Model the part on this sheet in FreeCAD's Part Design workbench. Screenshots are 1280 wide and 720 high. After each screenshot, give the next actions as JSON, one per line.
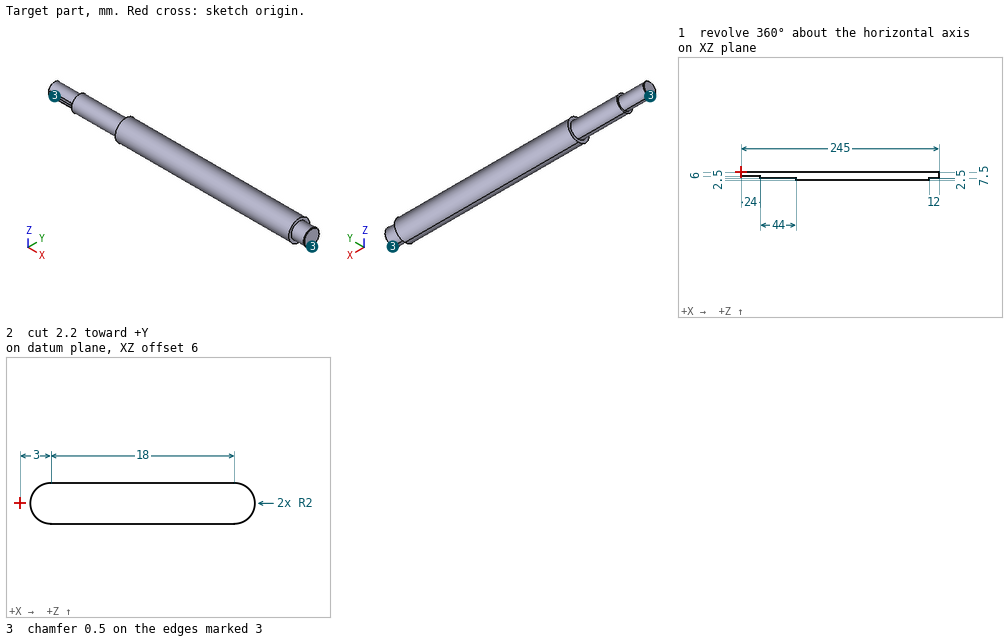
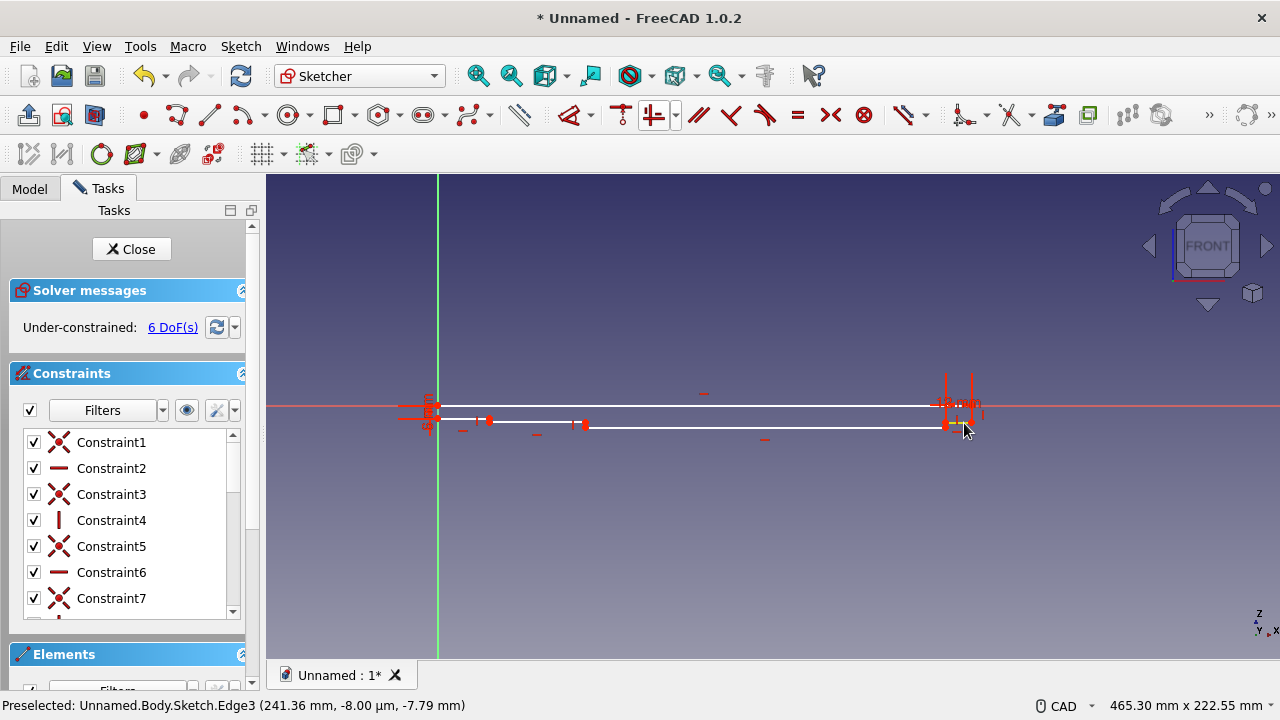
{"action": "left_click", "coordinate": [557, 422]}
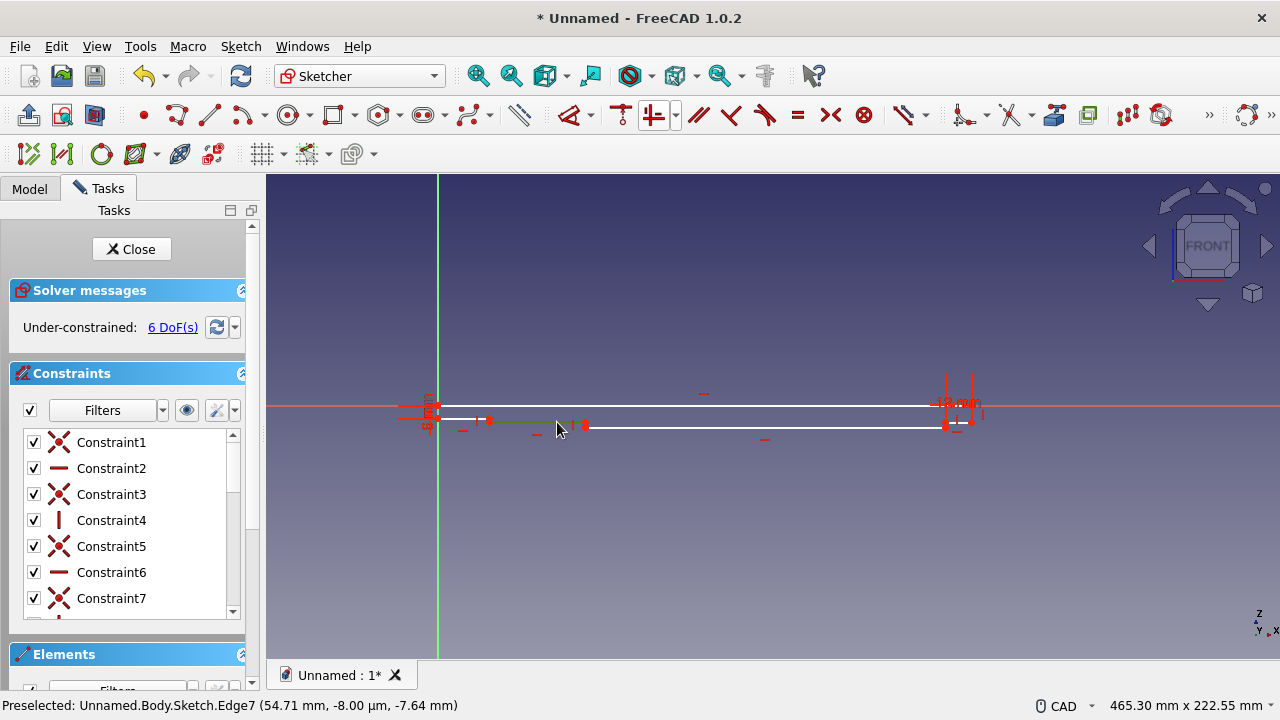
{"action": "left_click", "coordinate": [590, 116]}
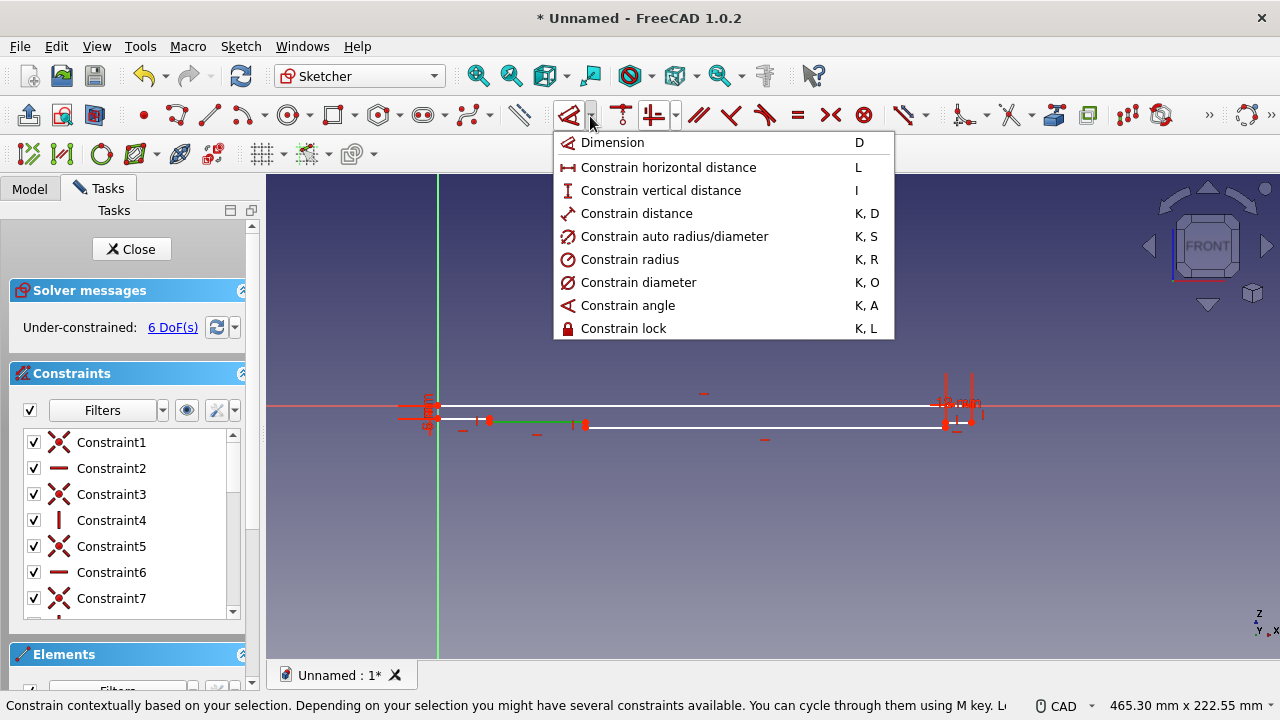
{"action": "left_click", "coordinate": [724, 168]}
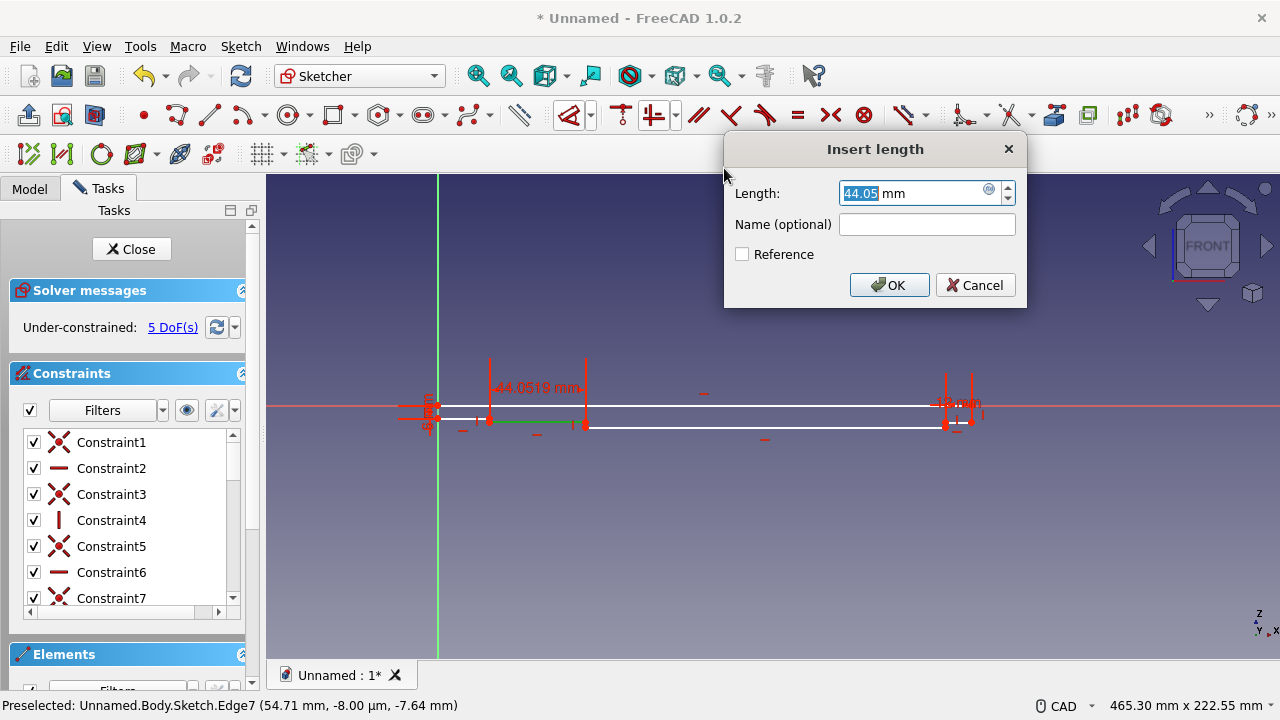
{"action": "type", "text": "44"}
{"action": "key", "text": "Return"}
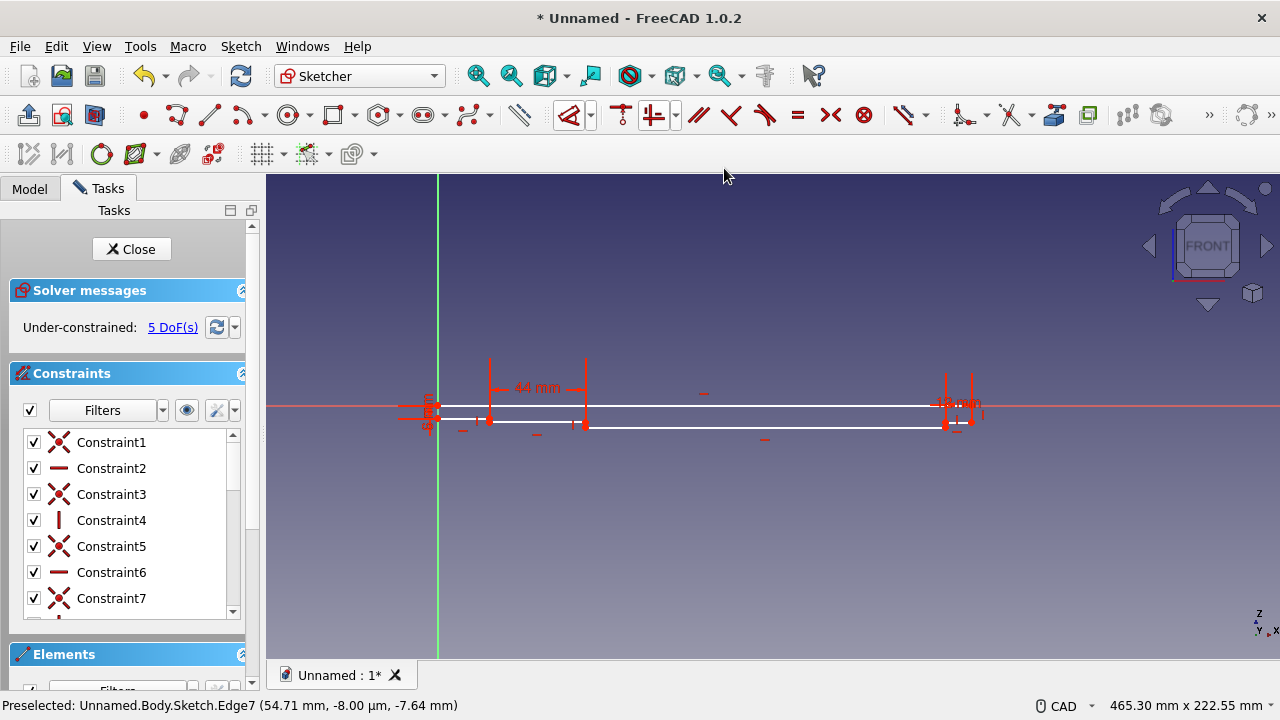
{"action": "left_click", "coordinate": [453, 419]}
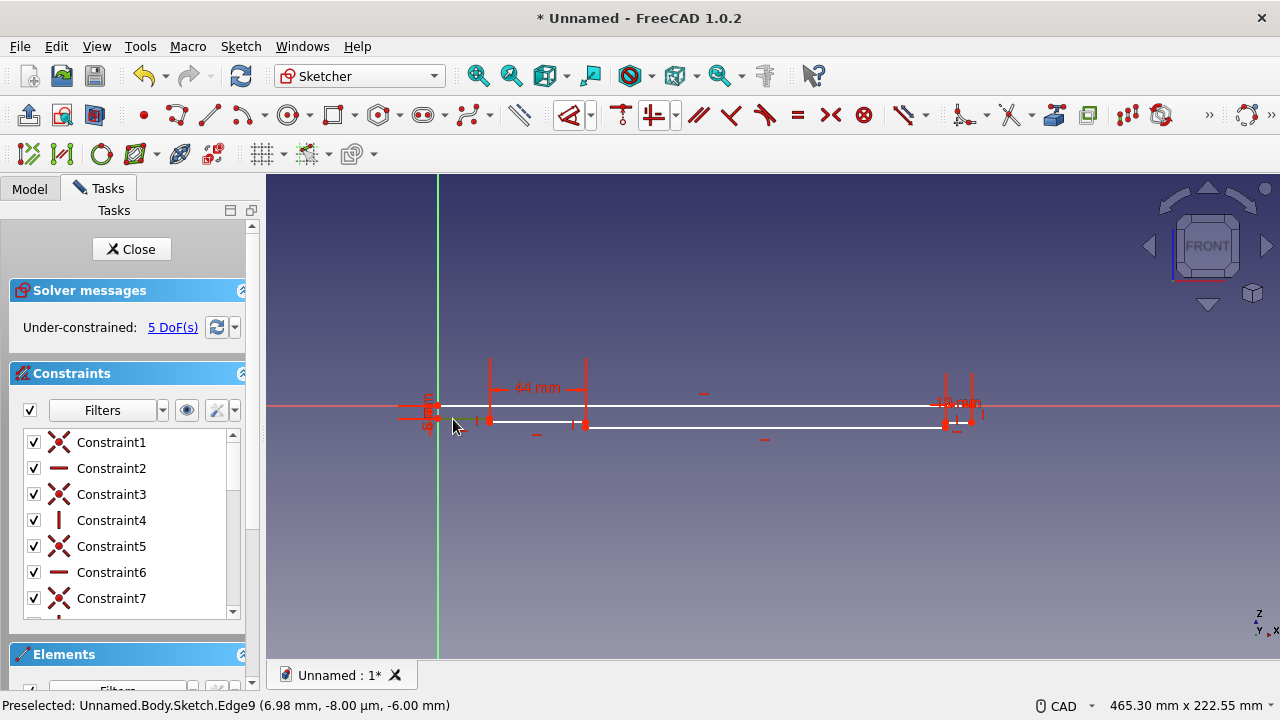
{"action": "left_click", "coordinate": [590, 116]}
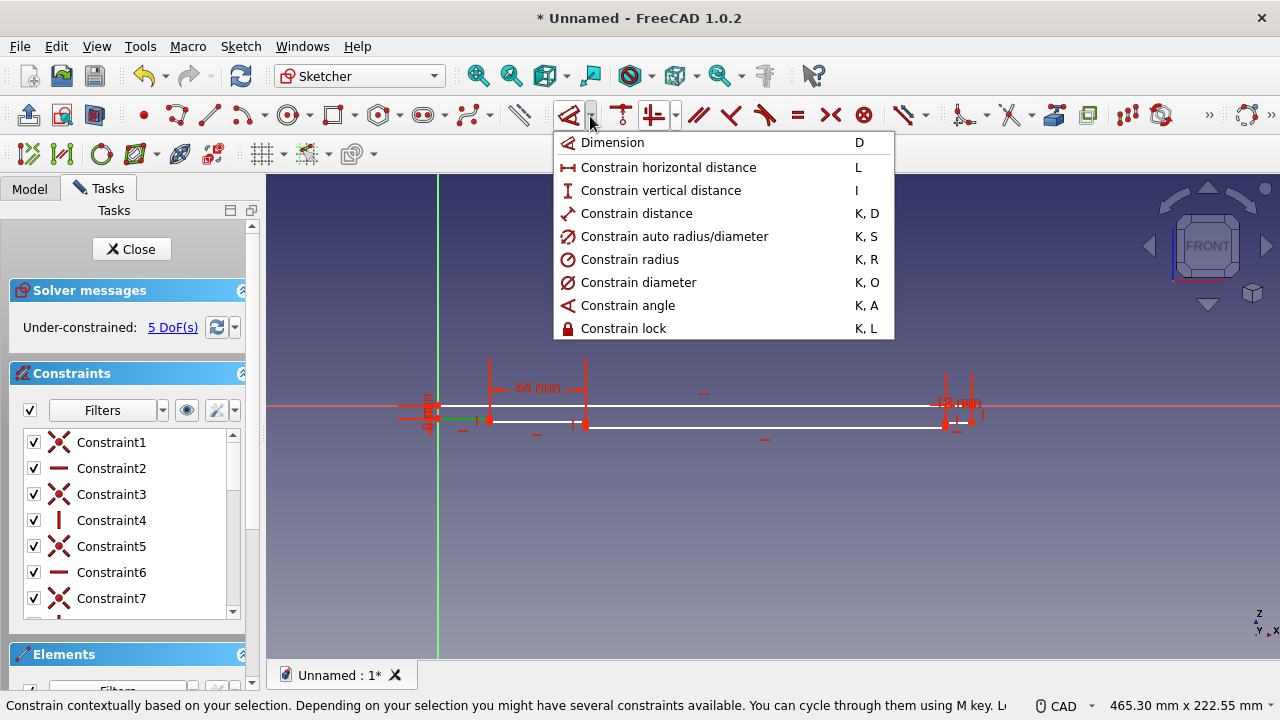
{"action": "left_click", "coordinate": [724, 168]}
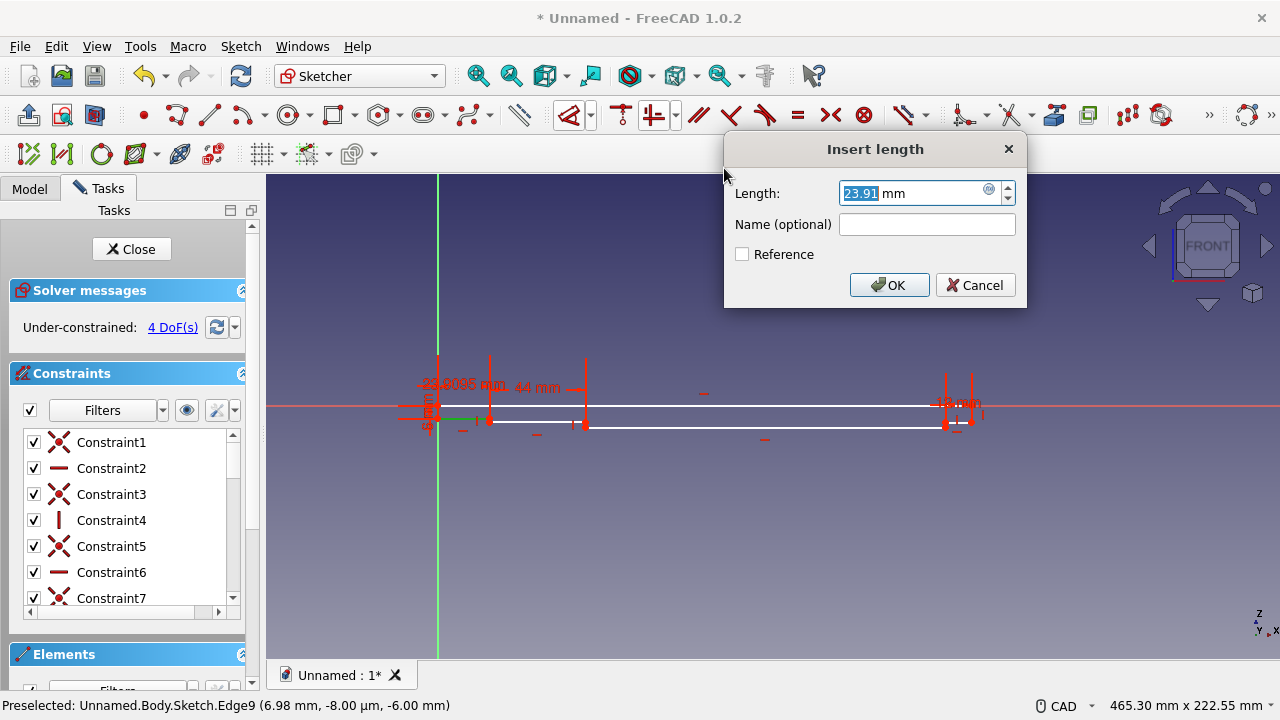
{"action": "type", "text": "24"}
{"action": "key", "text": "Return"}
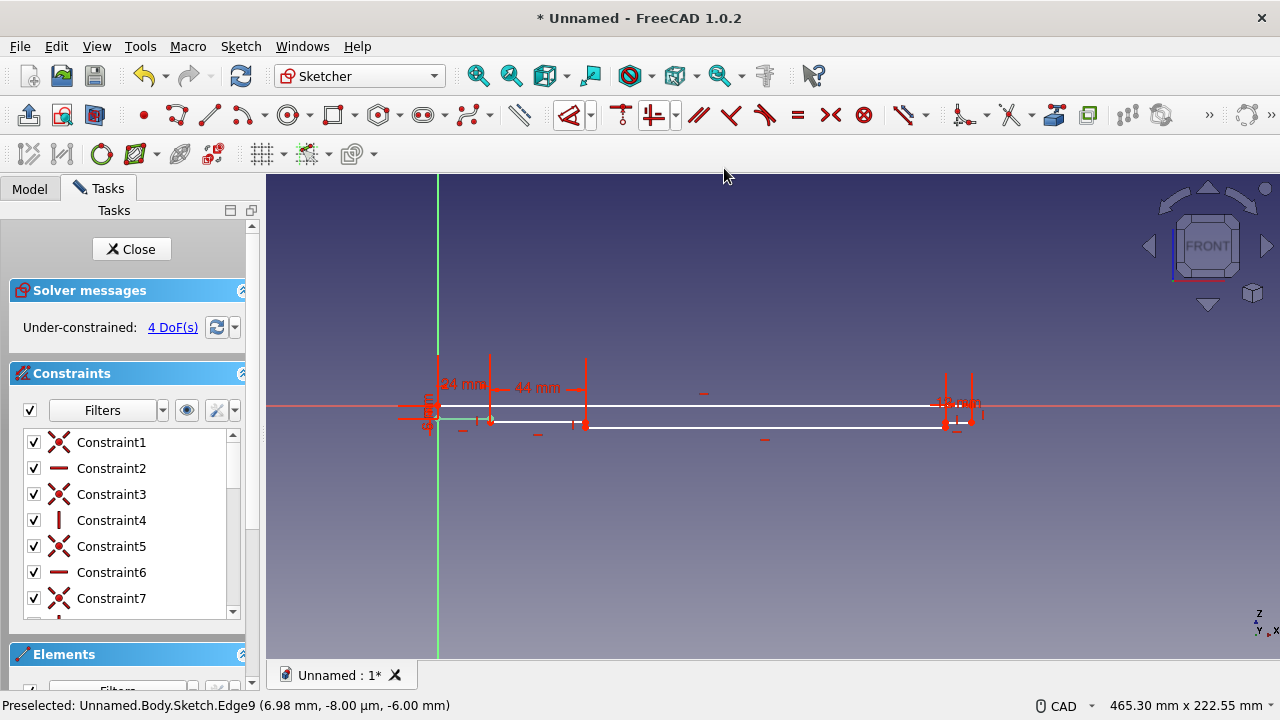
{"action": "left_click", "coordinate": [598, 406]}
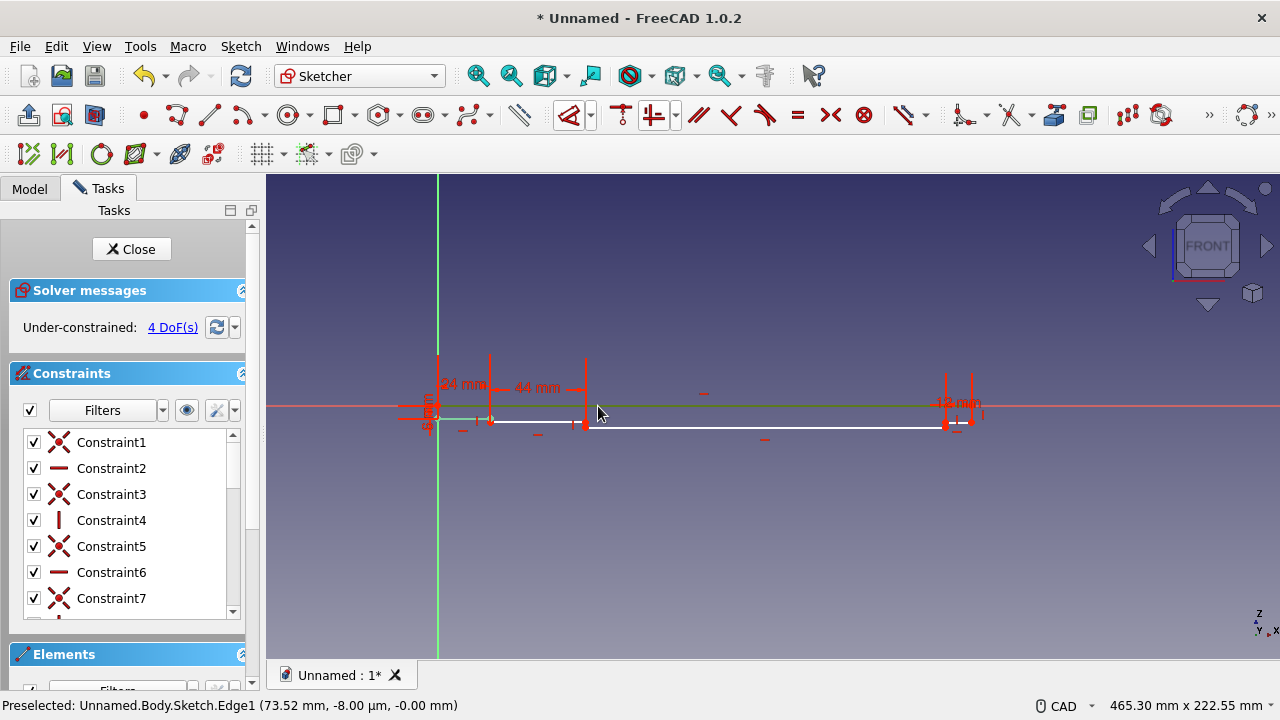
{"action": "left_click", "coordinate": [590, 116]}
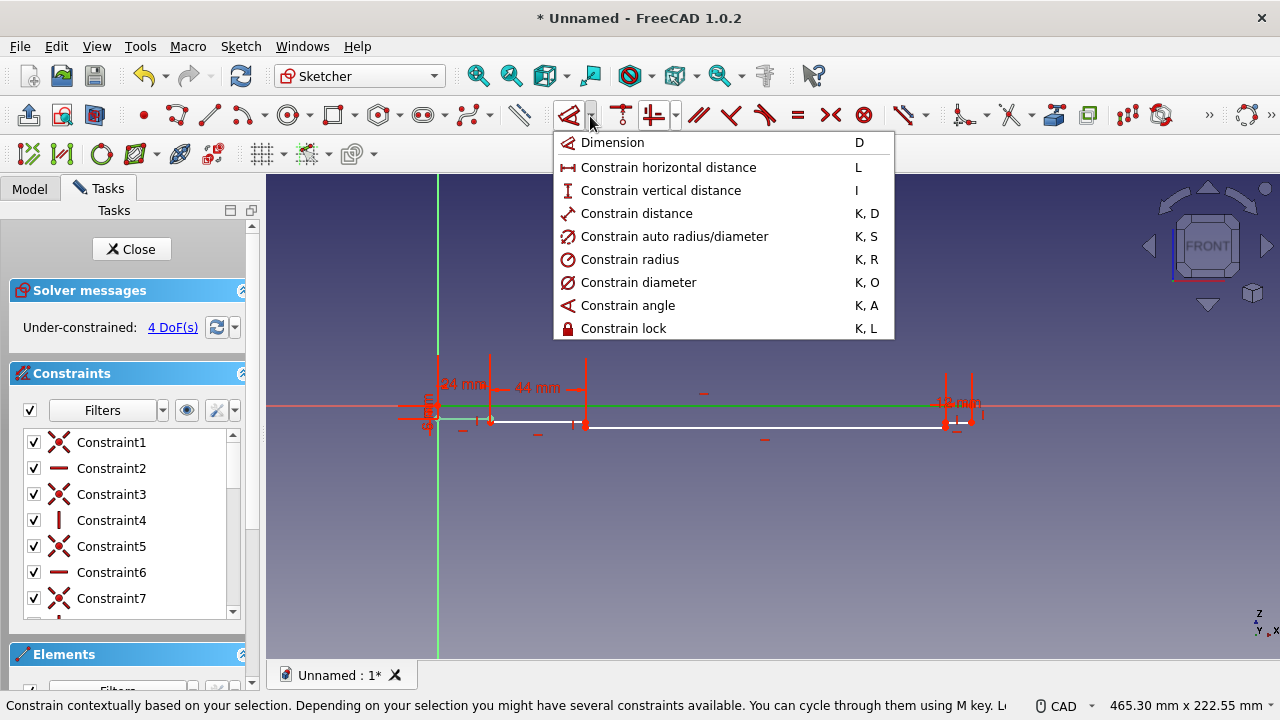
{"action": "left_click", "coordinate": [724, 168]}